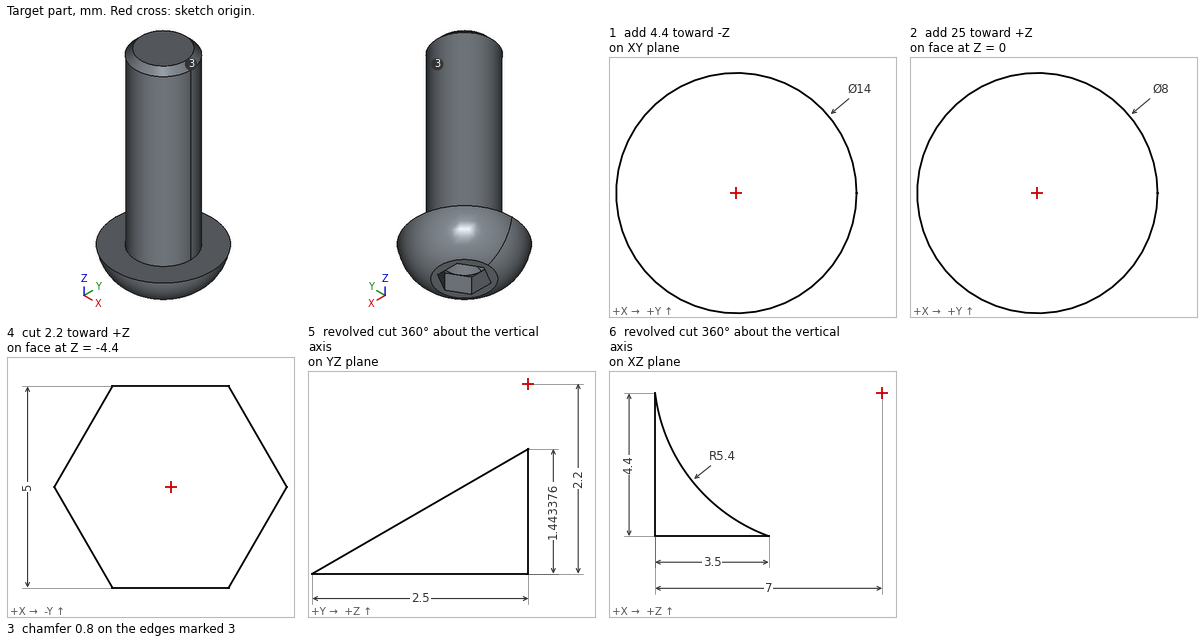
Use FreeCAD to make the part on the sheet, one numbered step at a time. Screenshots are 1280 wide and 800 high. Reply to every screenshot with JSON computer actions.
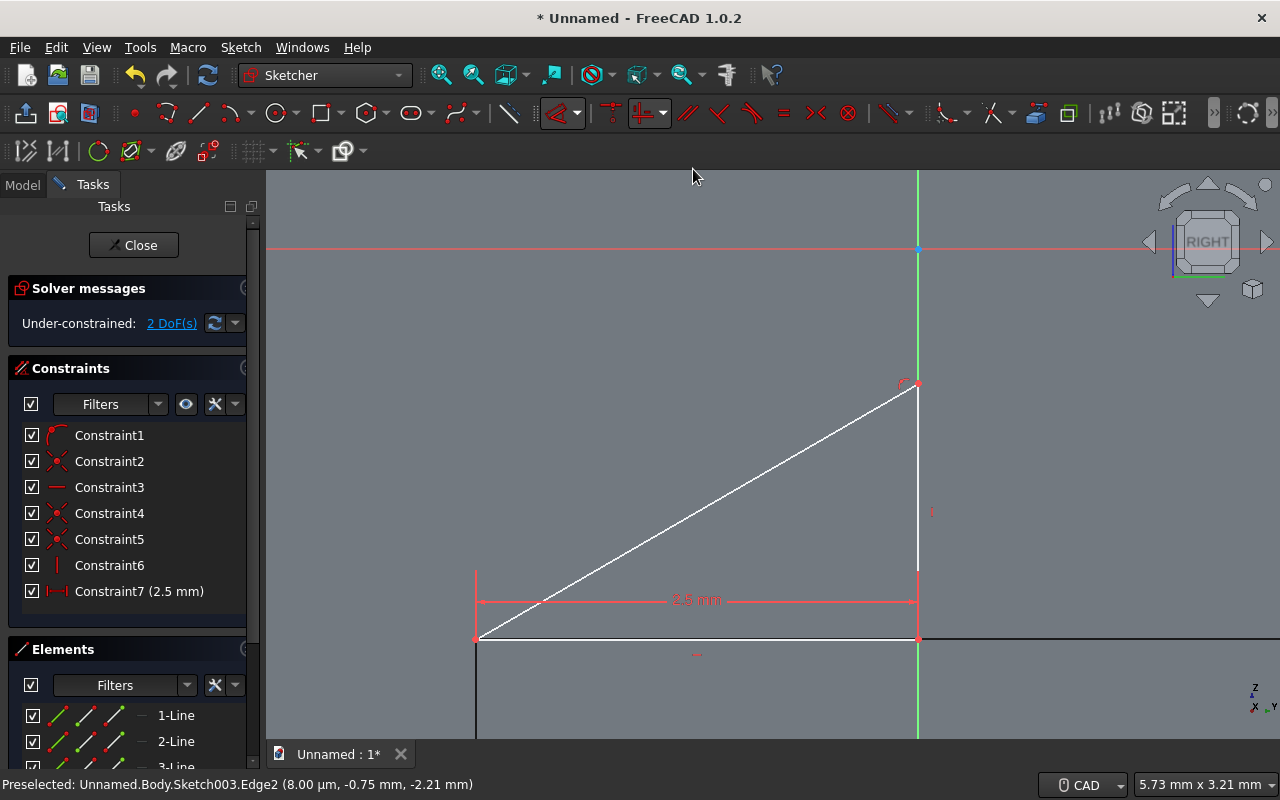
{"action": "left_click", "coordinate": [918, 640]}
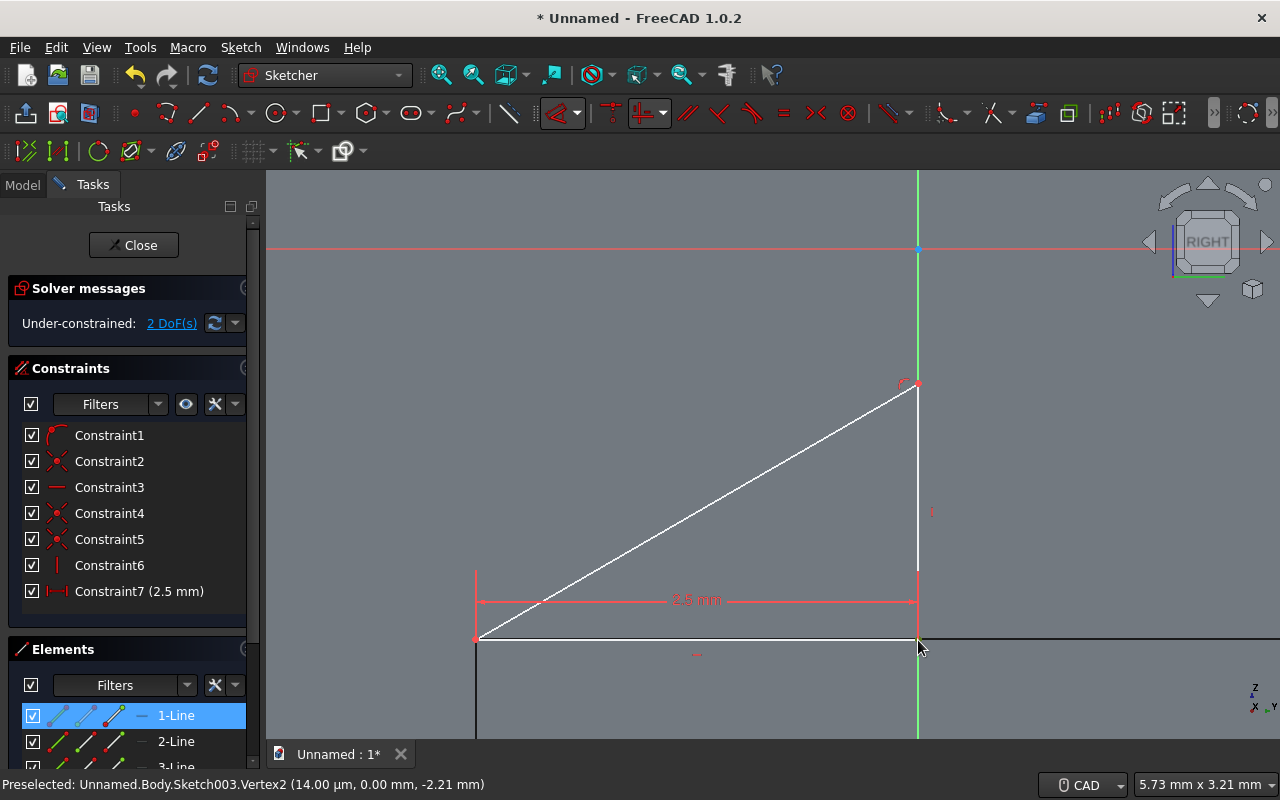
{"action": "key", "text": "i"}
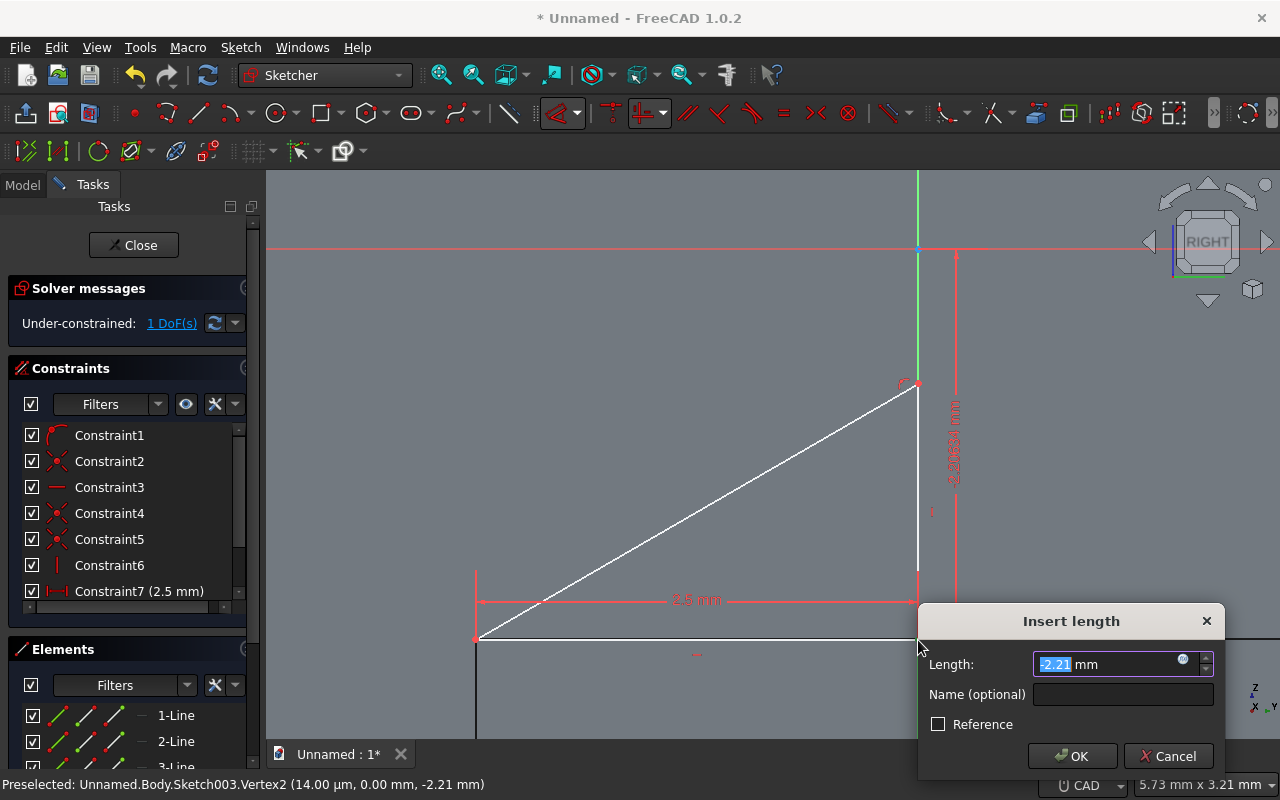
{"action": "type", "text": "-2.2"}
{"action": "key", "text": "Return"}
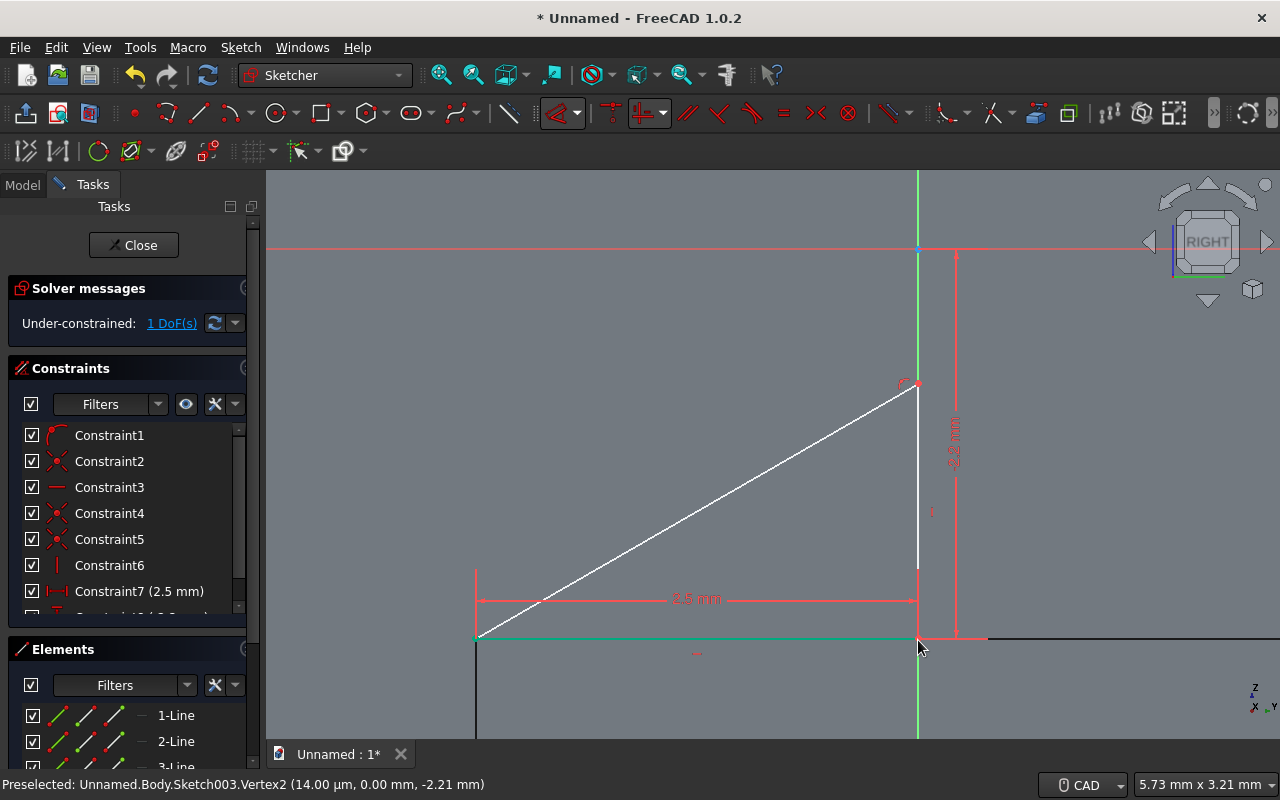
{"action": "left_click", "coordinate": [918, 460]}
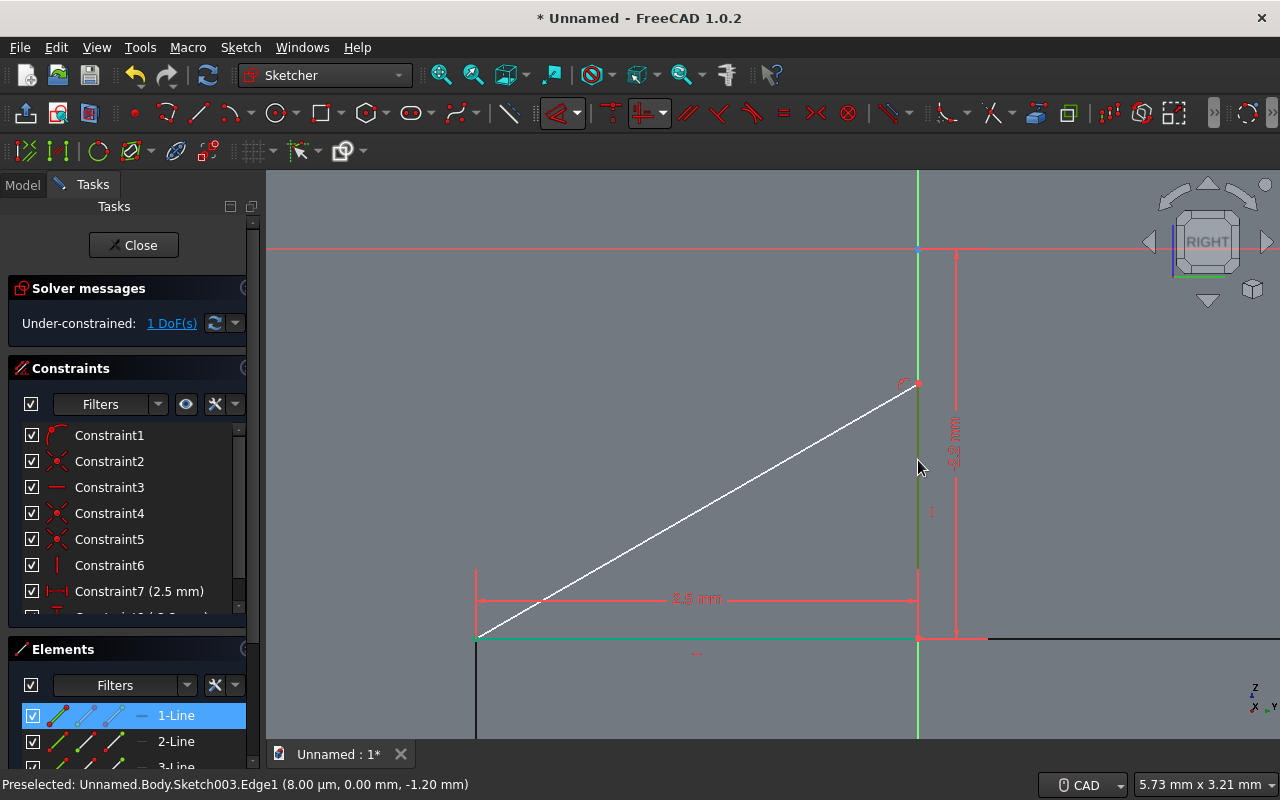
{"action": "left_click", "coordinate": [580, 114]}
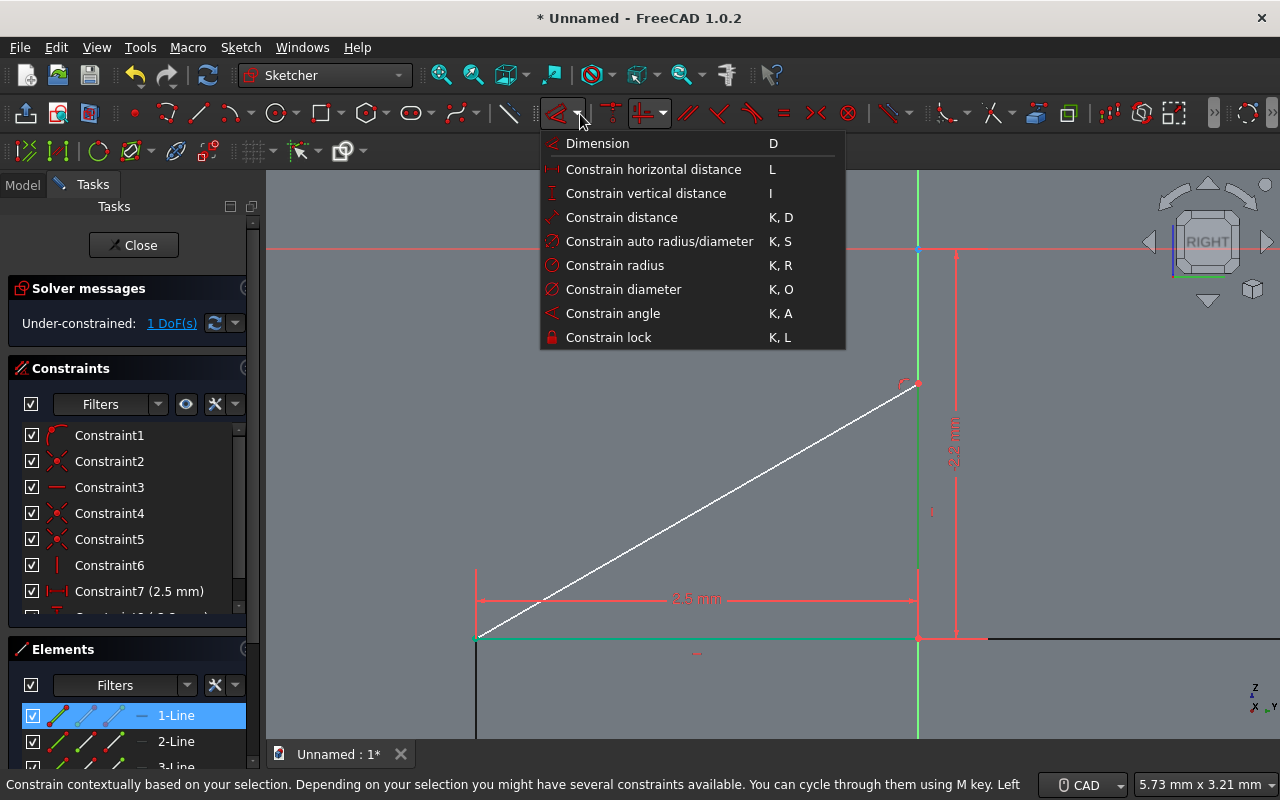
{"action": "left_click", "coordinate": [693, 193]}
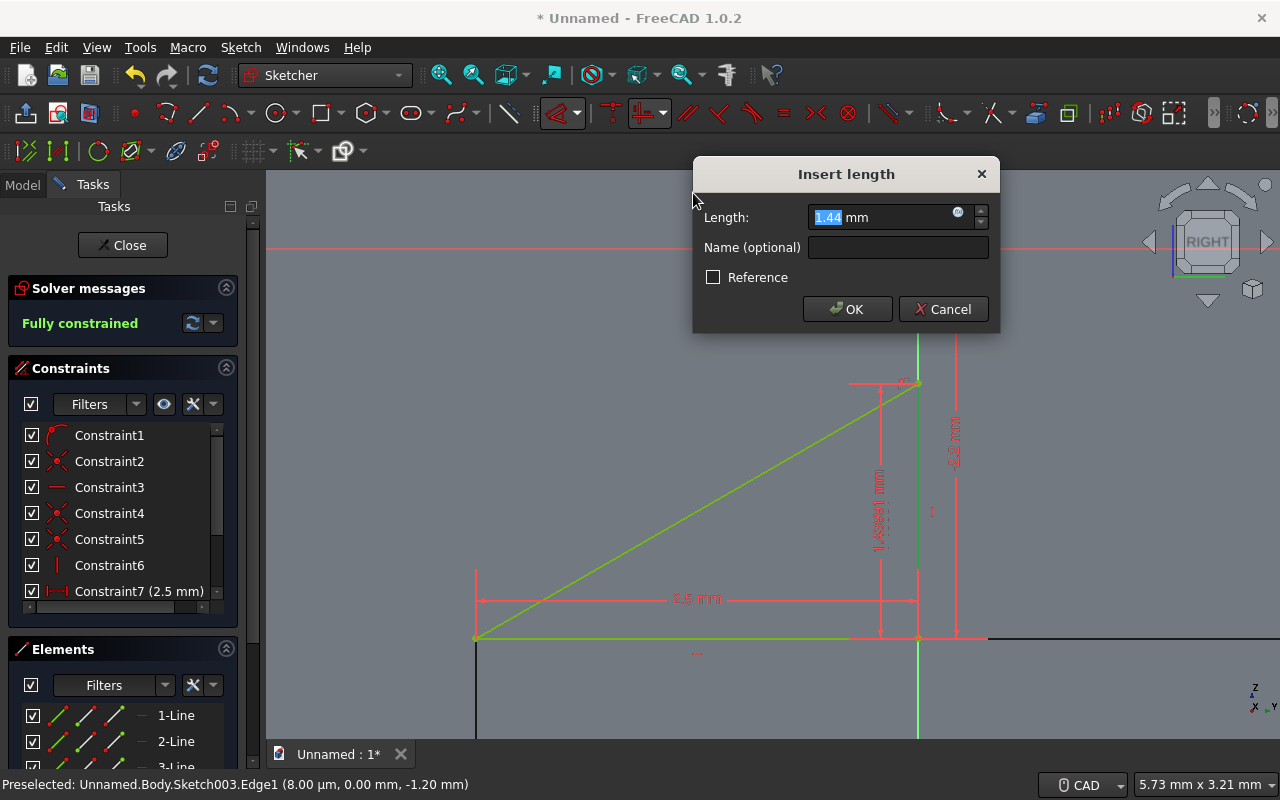
{"action": "type", "text": "1.443376"}
{"action": "key", "text": "Return"}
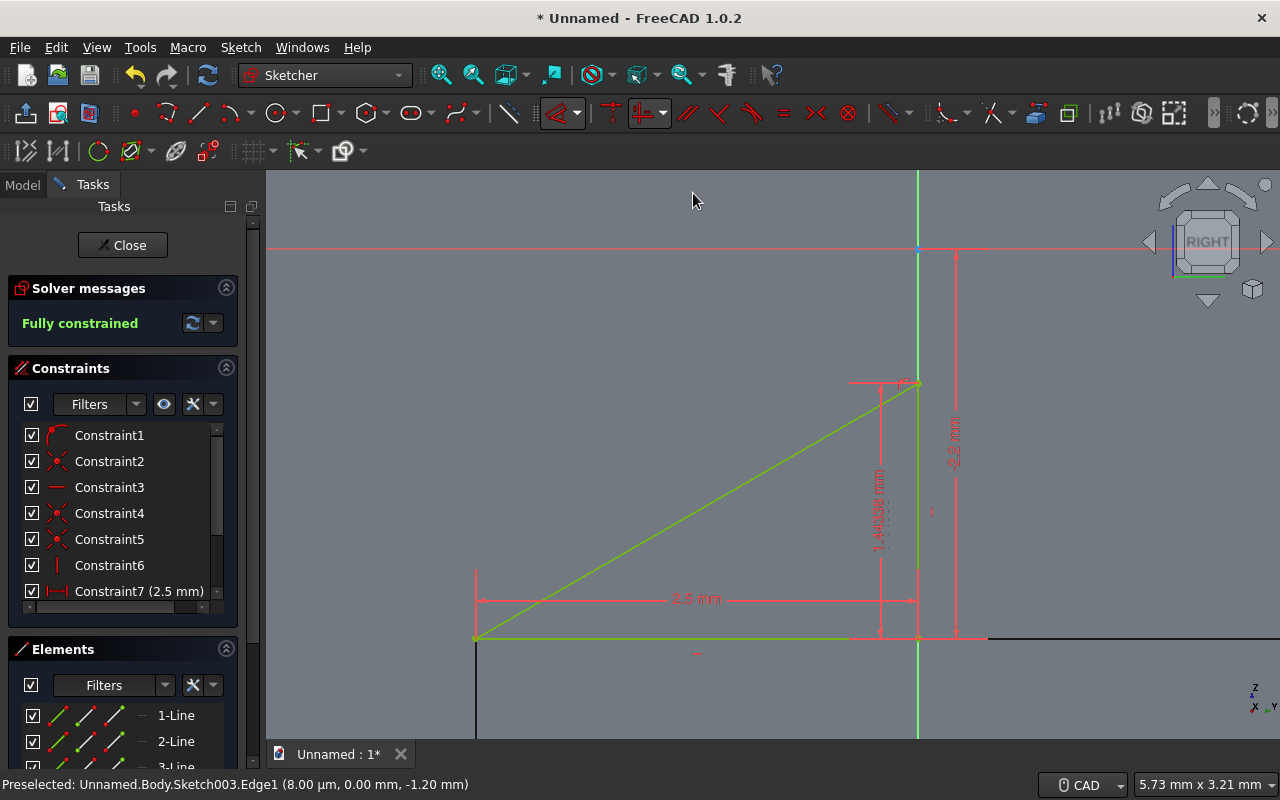
{"action": "left_click", "coordinate": [123, 245]}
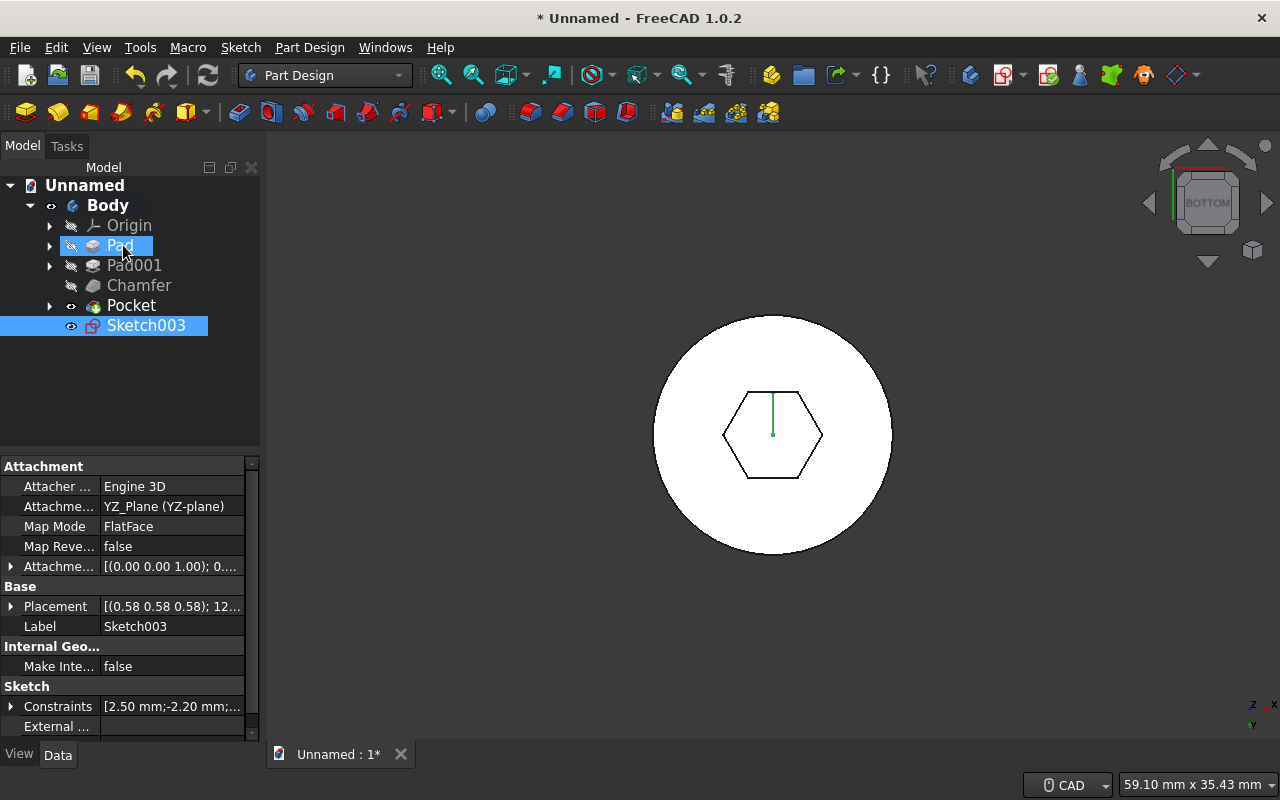
{"action": "left_click", "coordinate": [304, 112]}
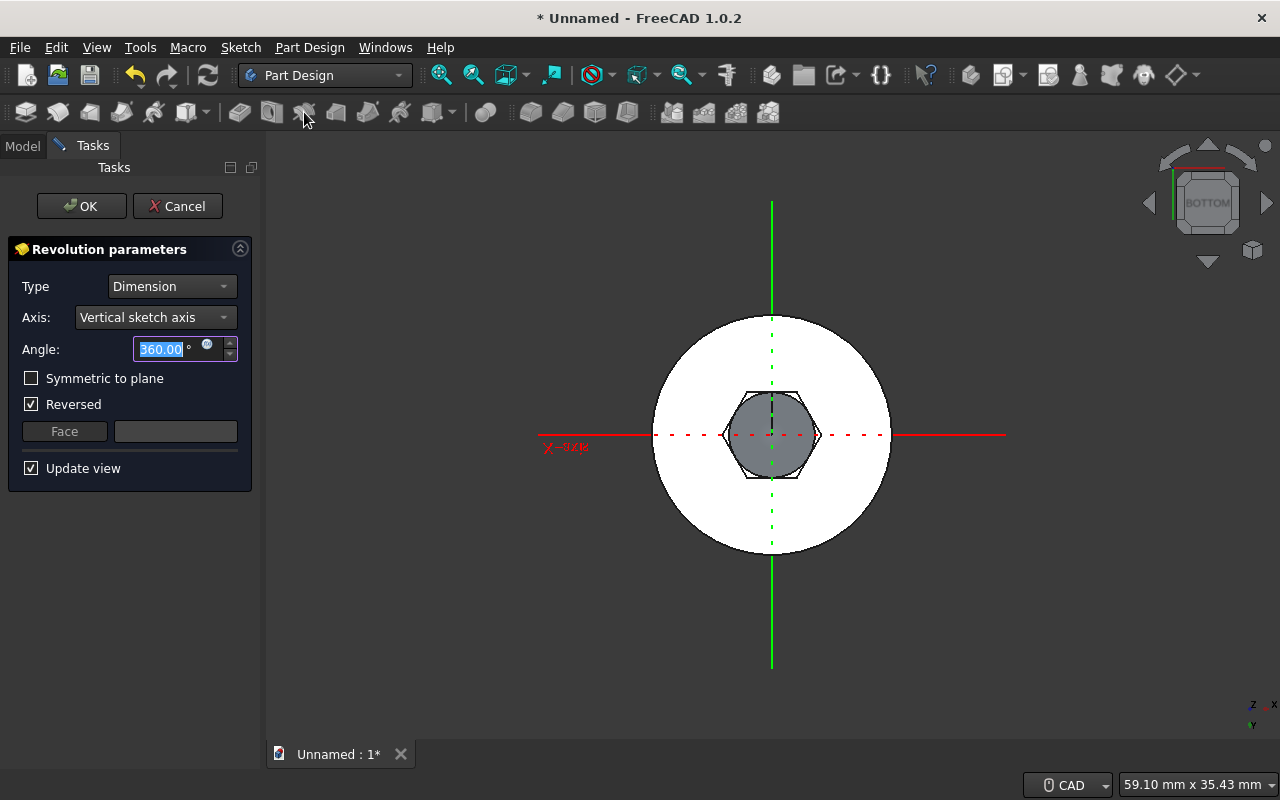
{"action": "left_click", "coordinate": [82, 206]}